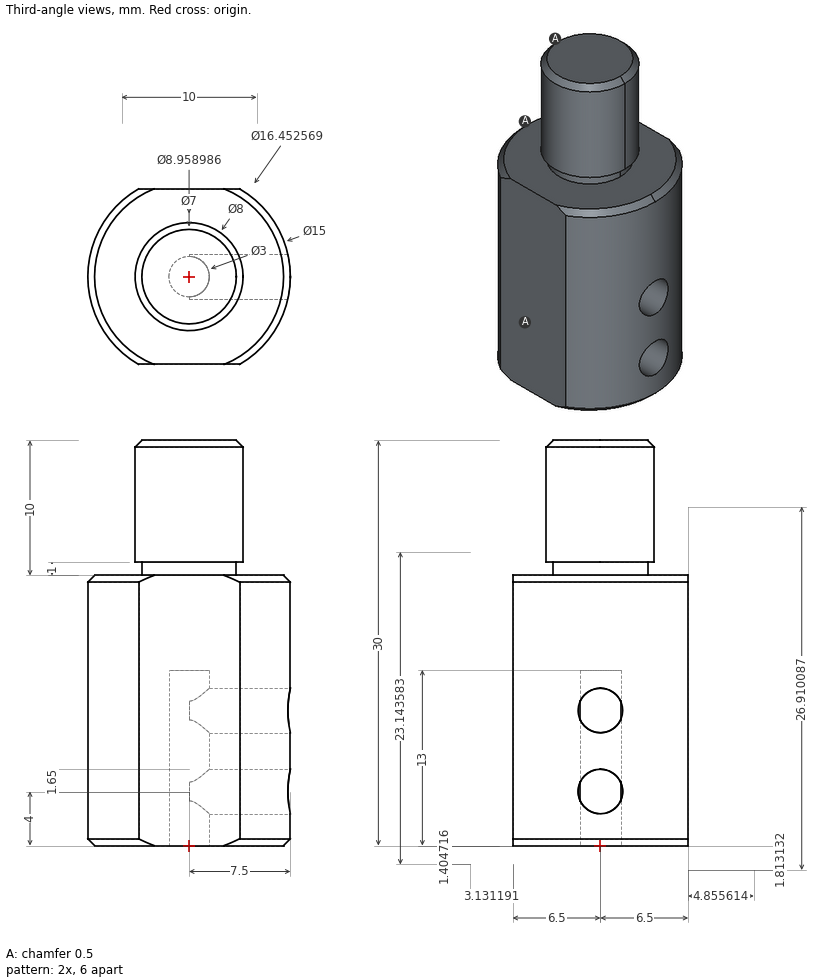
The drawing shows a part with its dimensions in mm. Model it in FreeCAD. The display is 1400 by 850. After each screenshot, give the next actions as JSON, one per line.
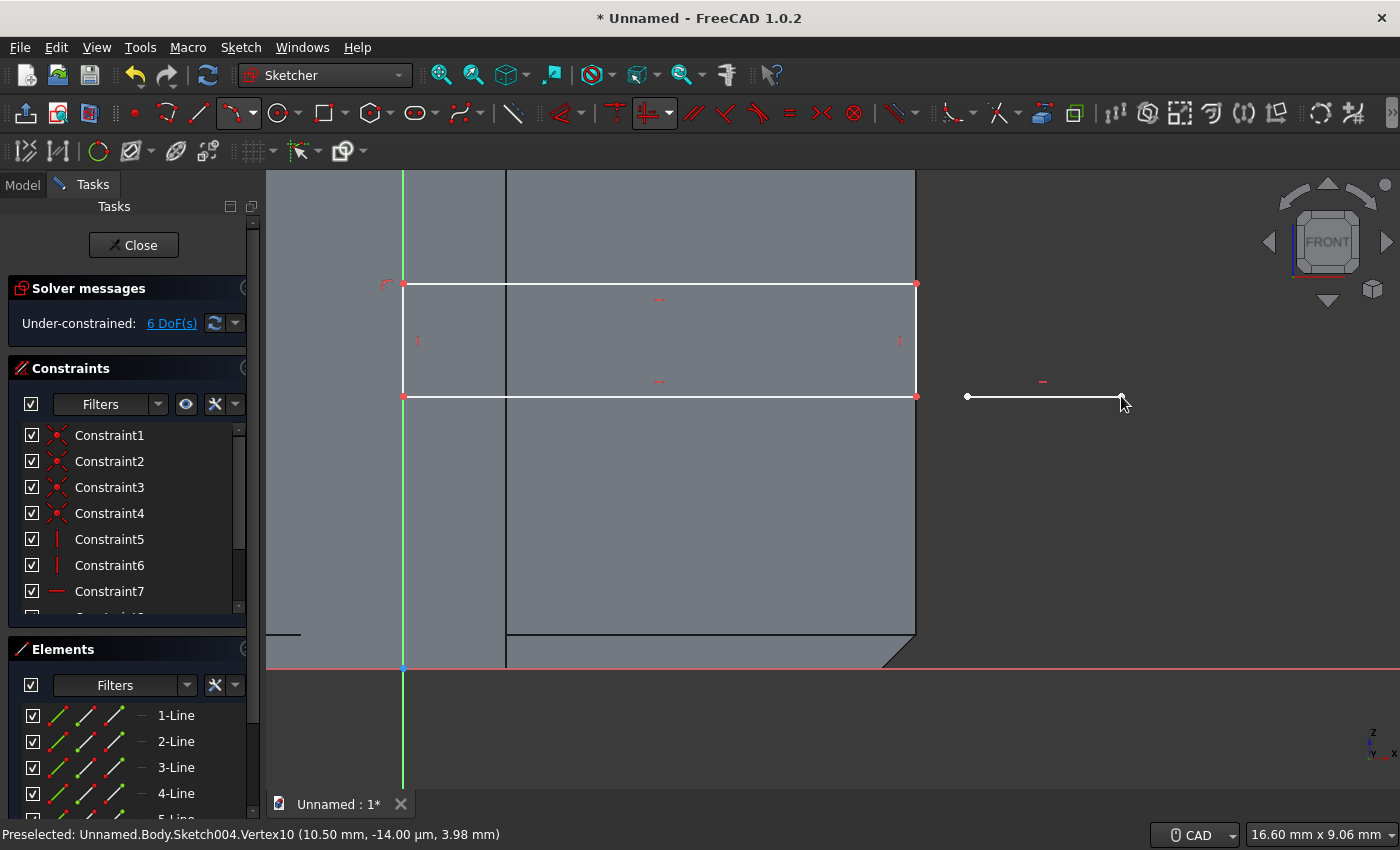
{"action": "left_click", "coordinate": [1013, 397]}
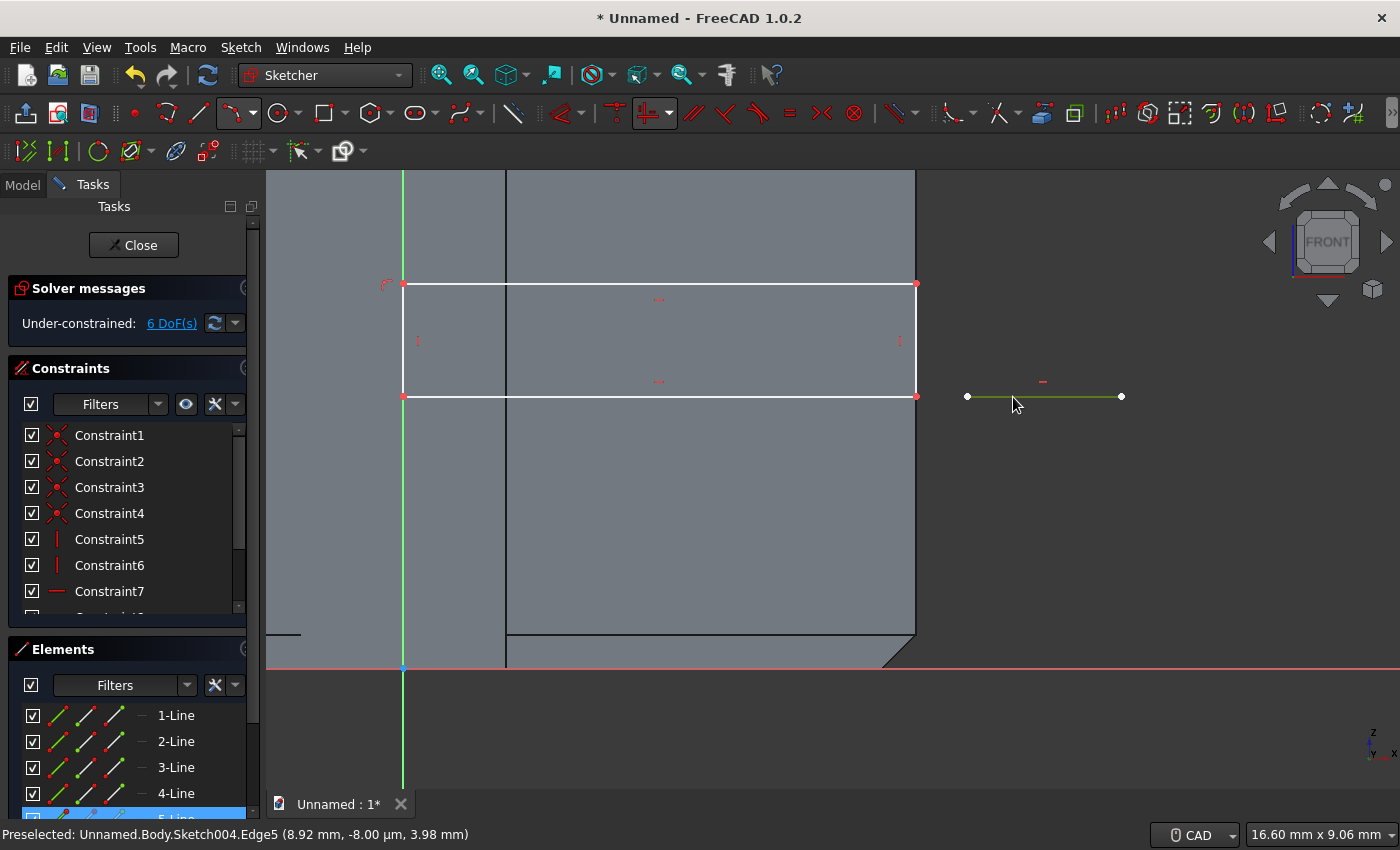
{"action": "left_click", "coordinate": [514, 114]}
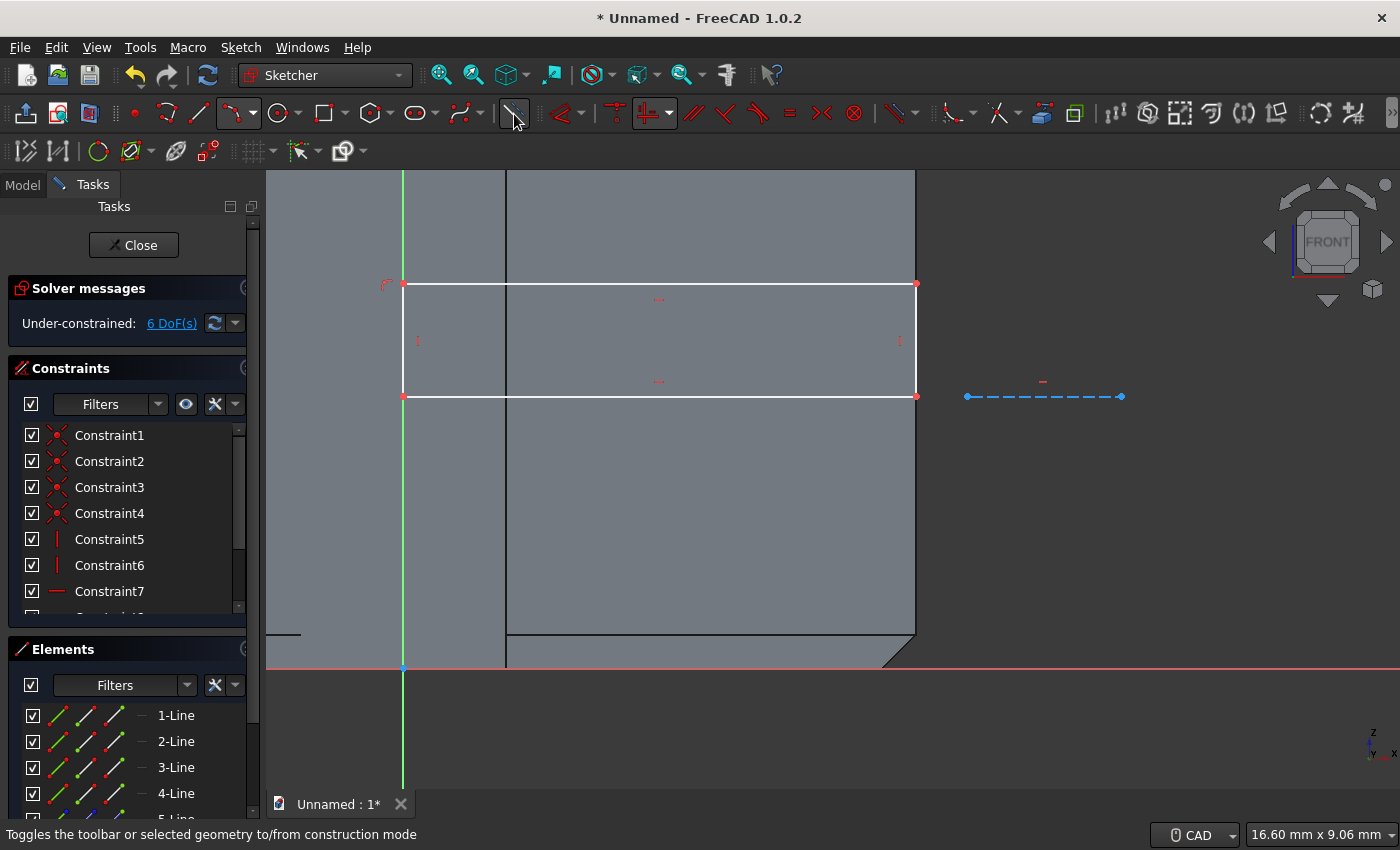
{"action": "left_click", "coordinate": [560, 114]}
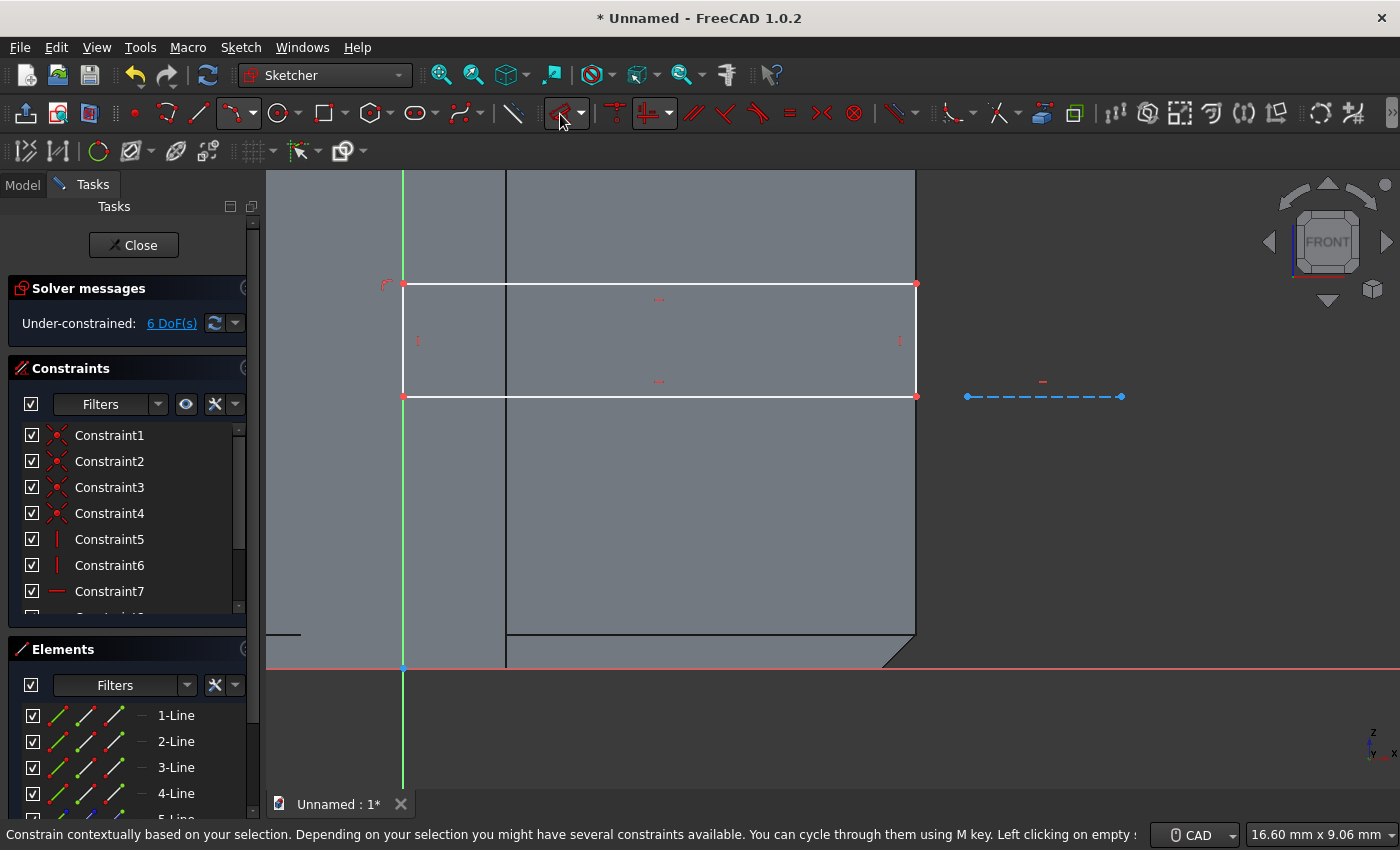
{"action": "left_click", "coordinate": [403, 397]}
{"action": "left_click", "coordinate": [369, 533]}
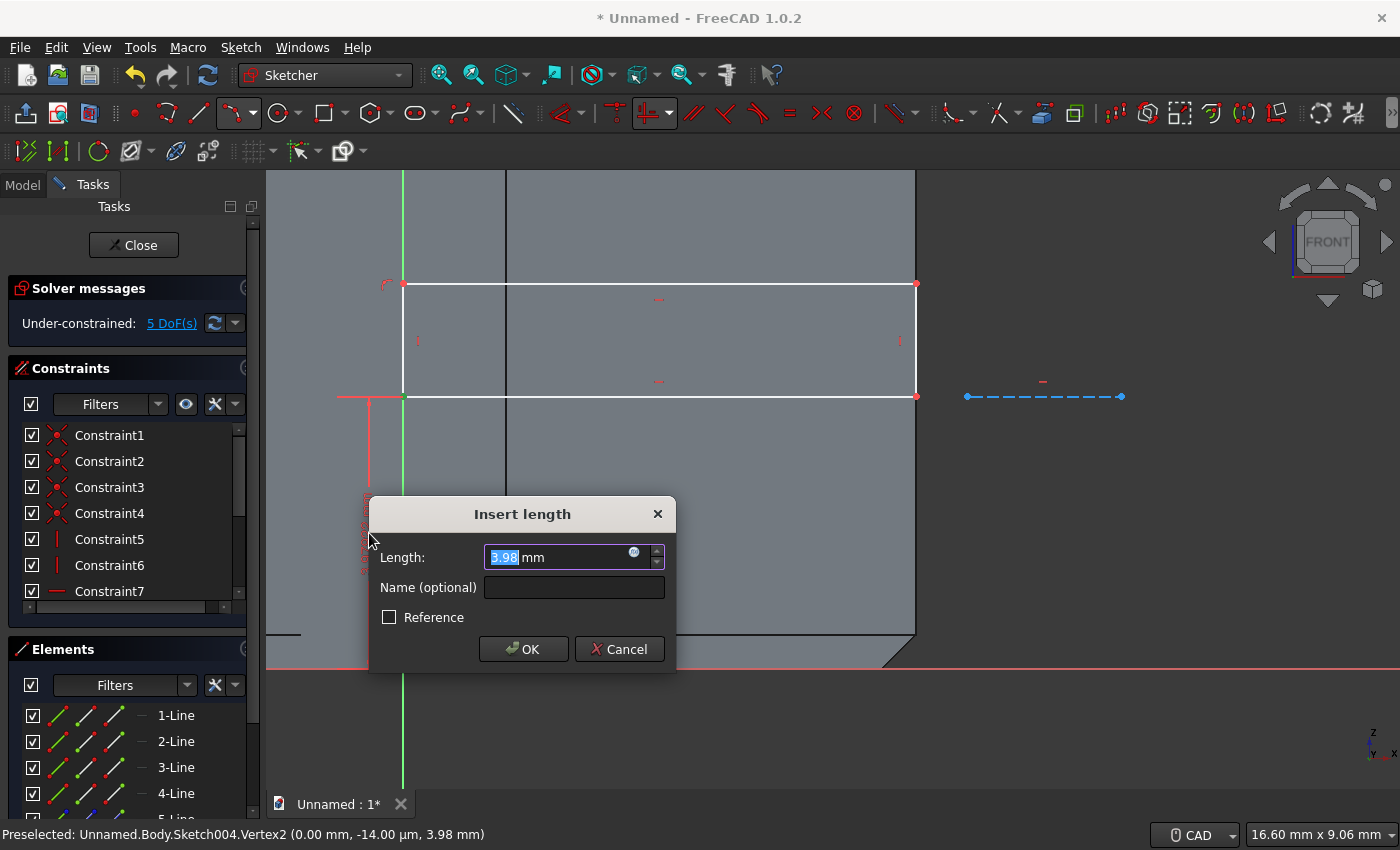
{"action": "type", "text": "4"}
{"action": "key", "text": "Return"}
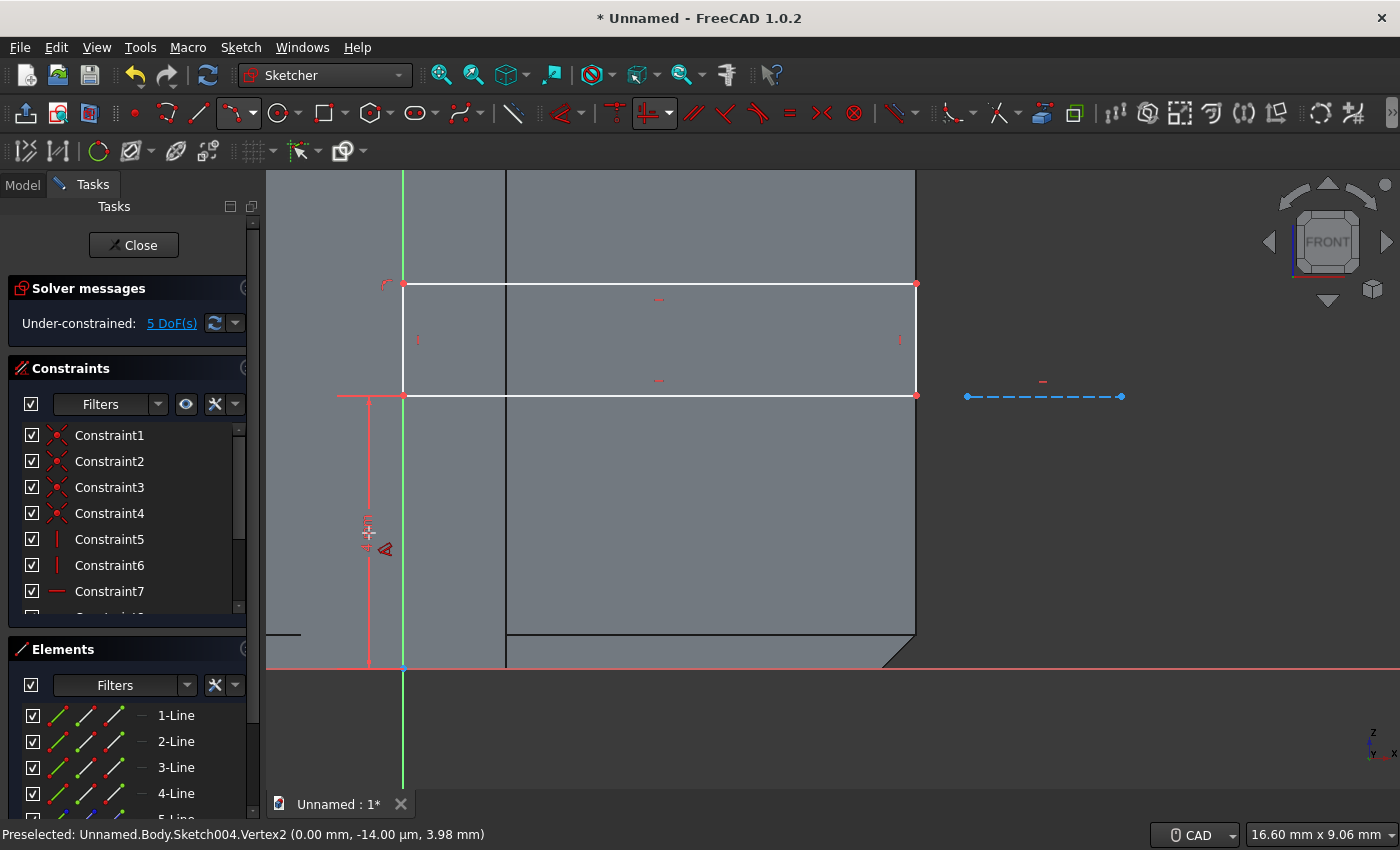
{"action": "left_click", "coordinate": [967, 397]}
{"action": "left_click", "coordinate": [369, 470]}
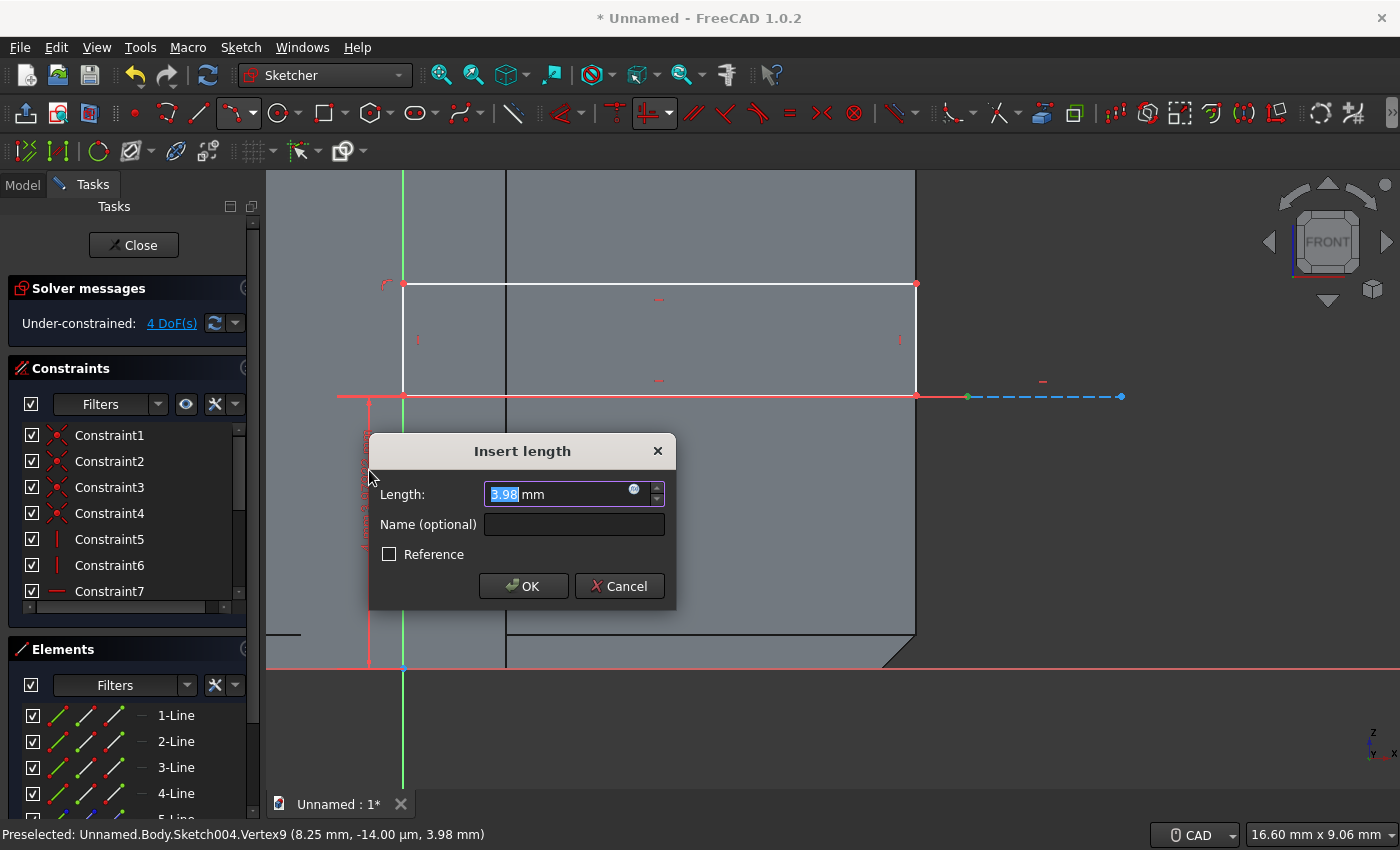
{"action": "type", "text": "4"}
{"action": "key", "text": "Return"}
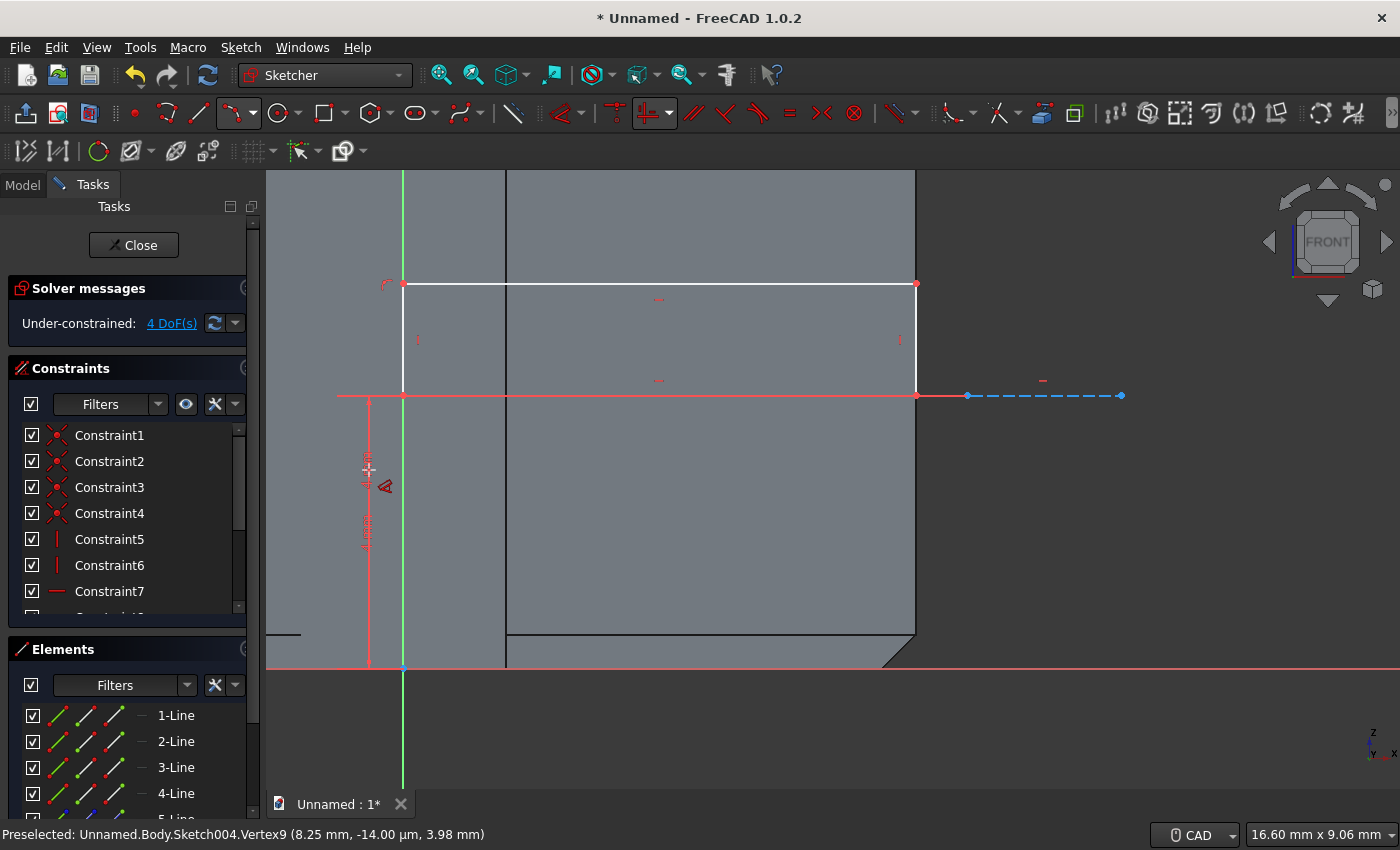
{"action": "left_click", "coordinate": [557, 396]}
{"action": "left_click", "coordinate": [660, 362]}